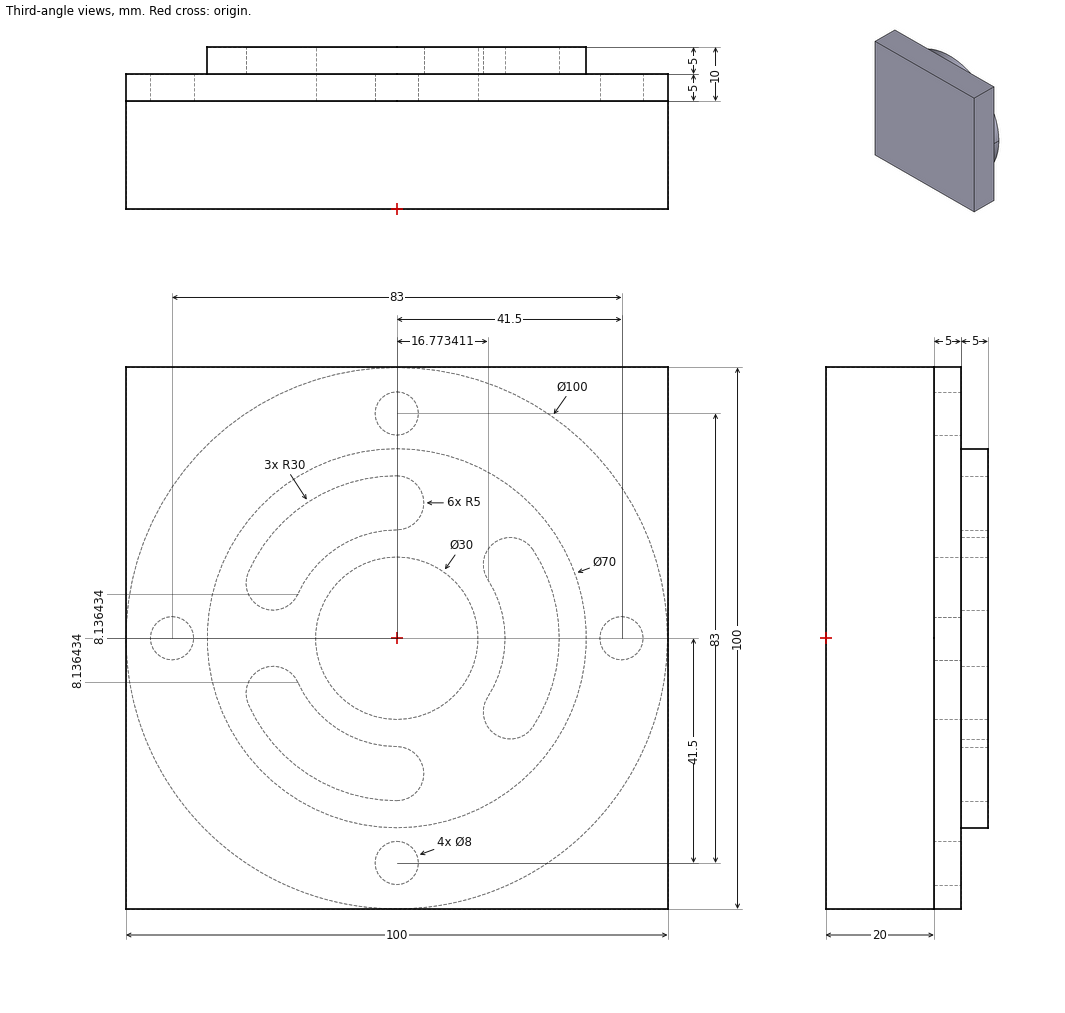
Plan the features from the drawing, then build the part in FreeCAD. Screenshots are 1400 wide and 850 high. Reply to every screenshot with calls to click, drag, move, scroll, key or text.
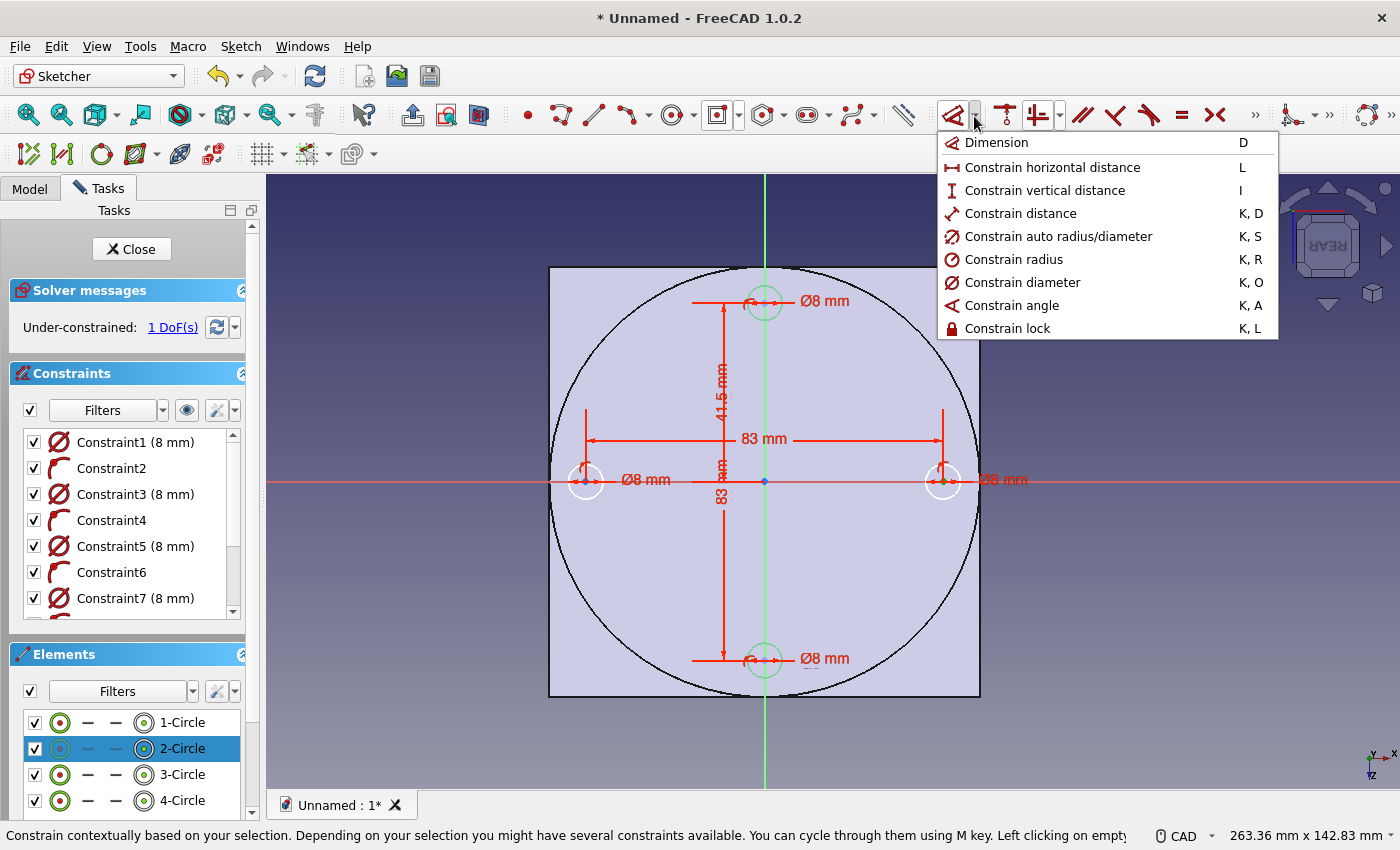
click(1108, 168)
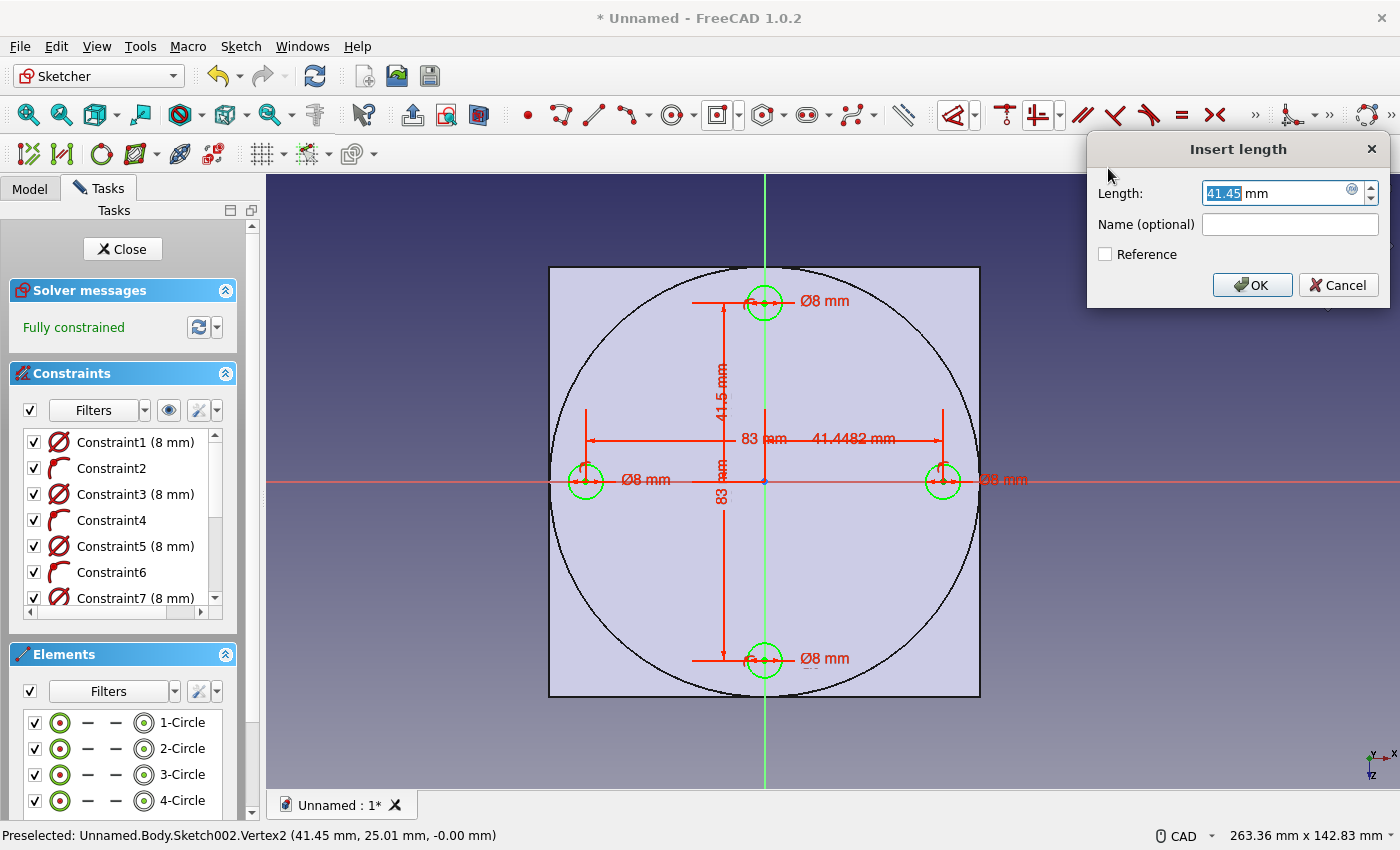
text(41.5)
key(Return)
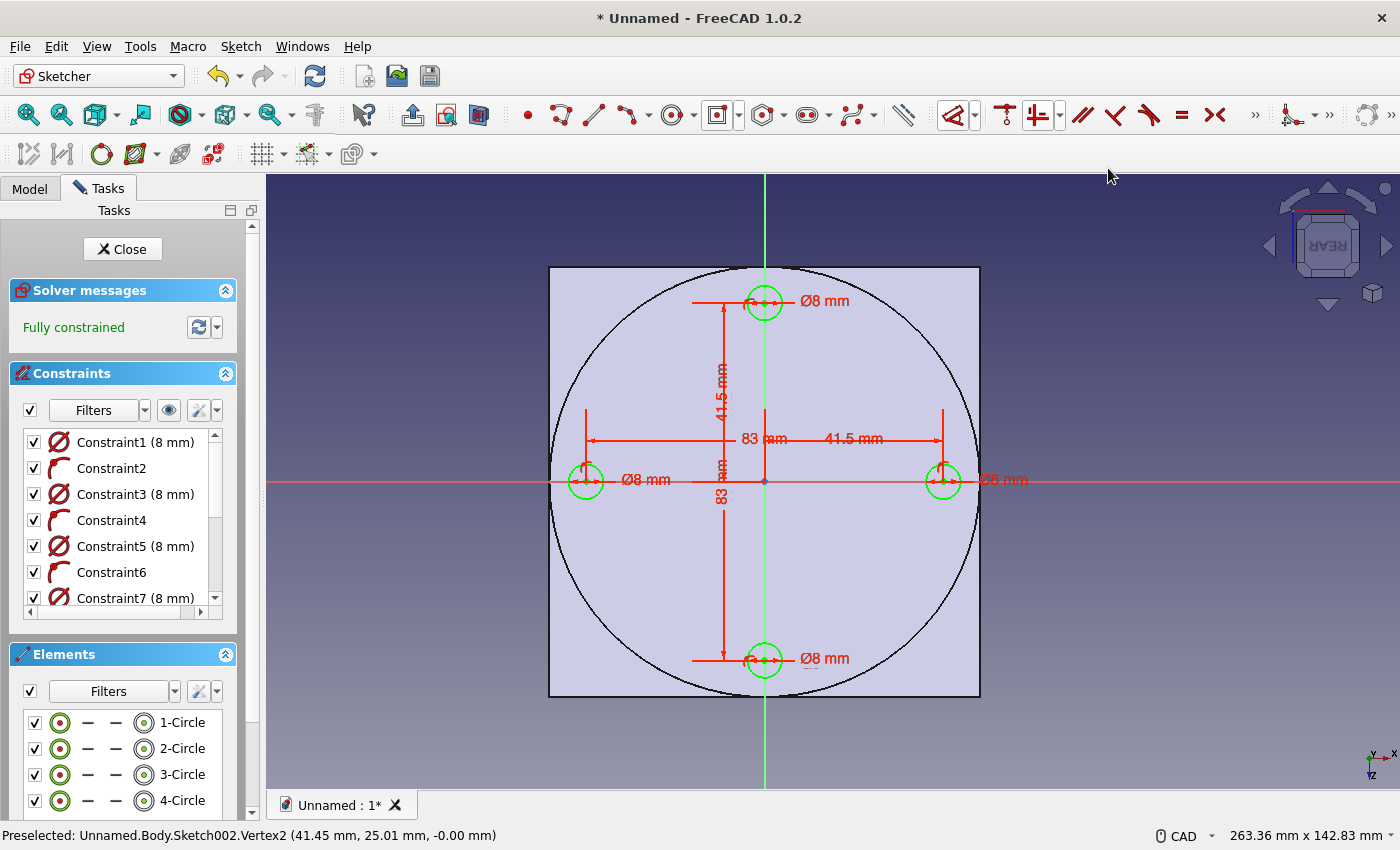
click(123, 249)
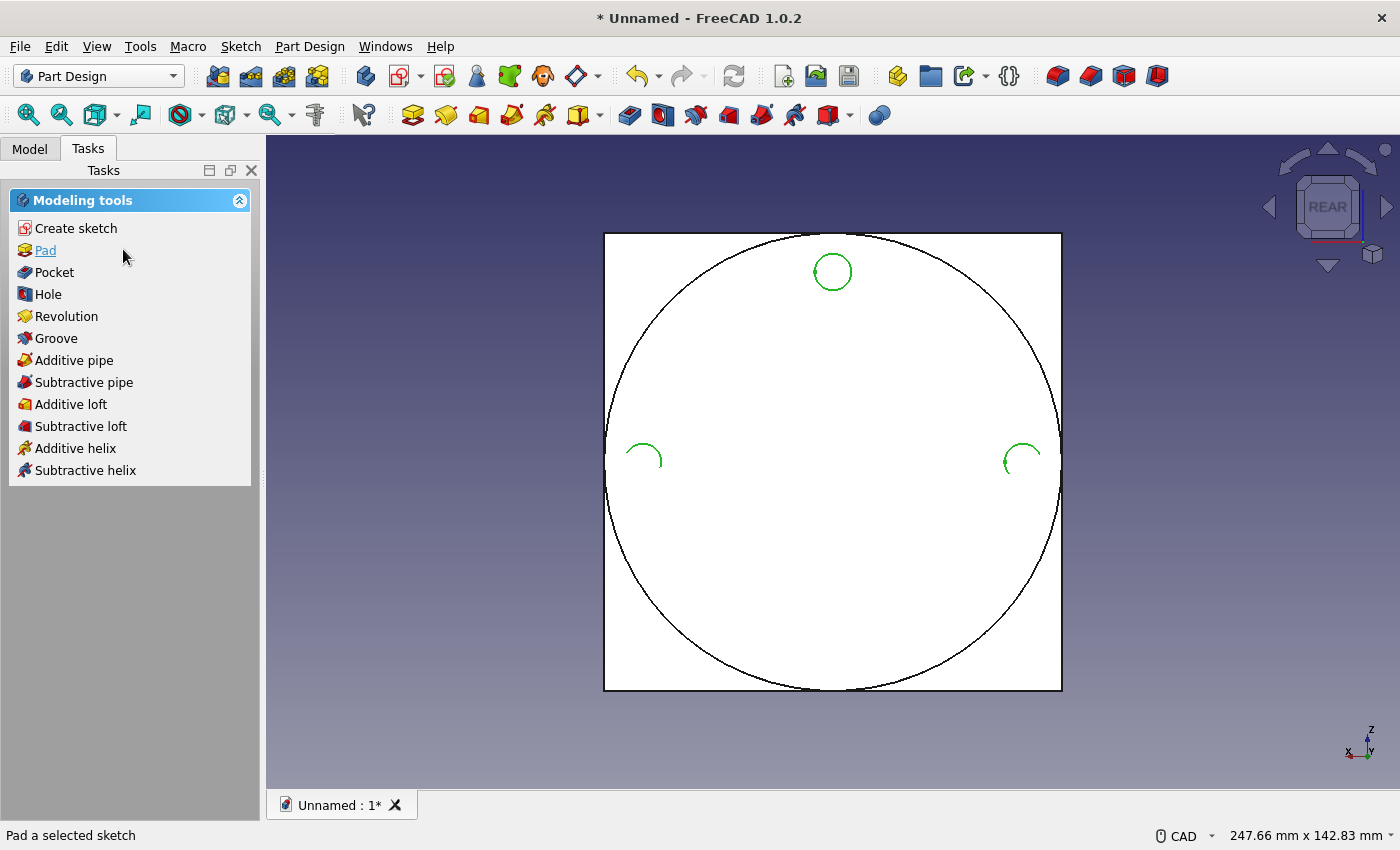
click(630, 116)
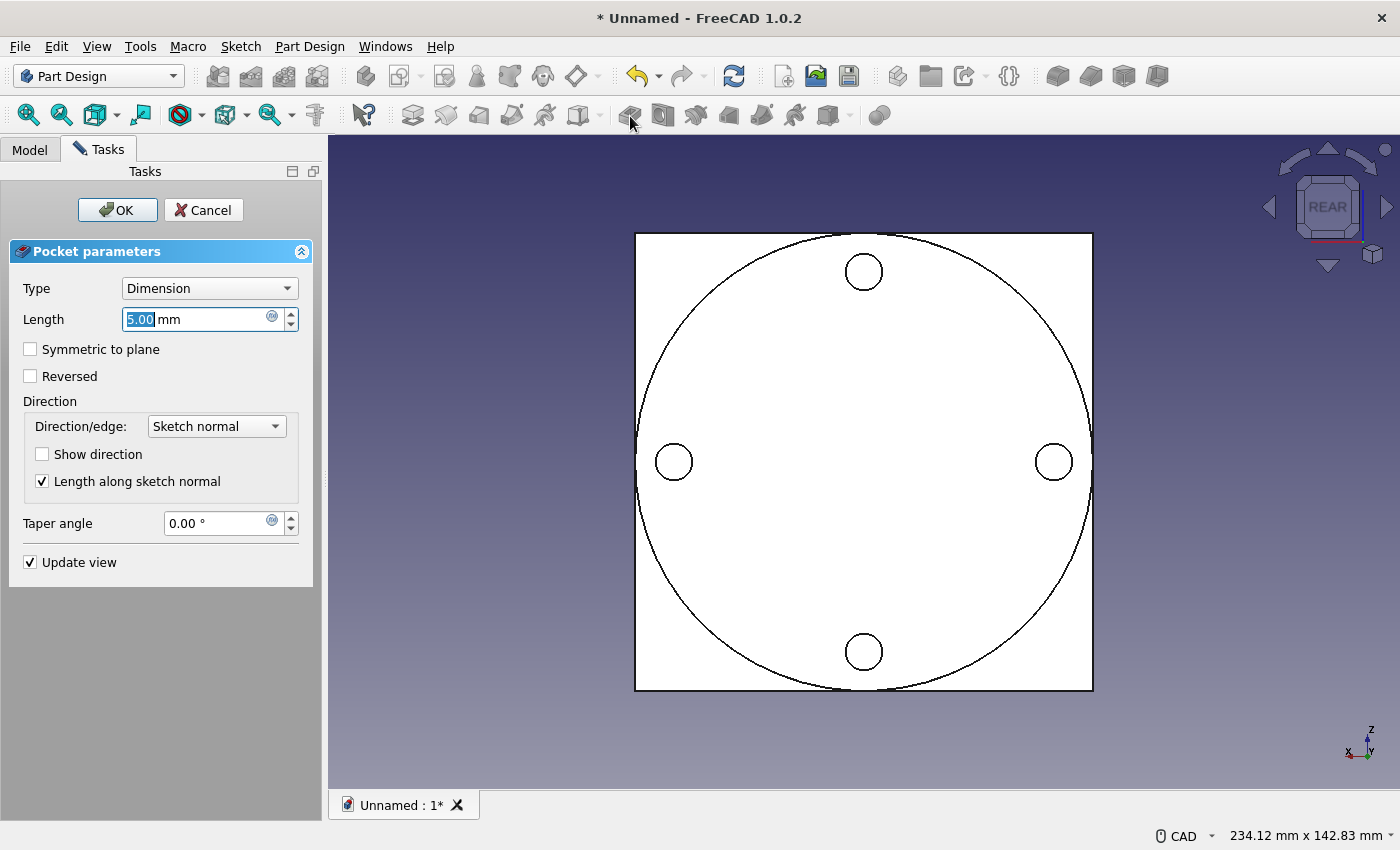
text(5)
key(Tab)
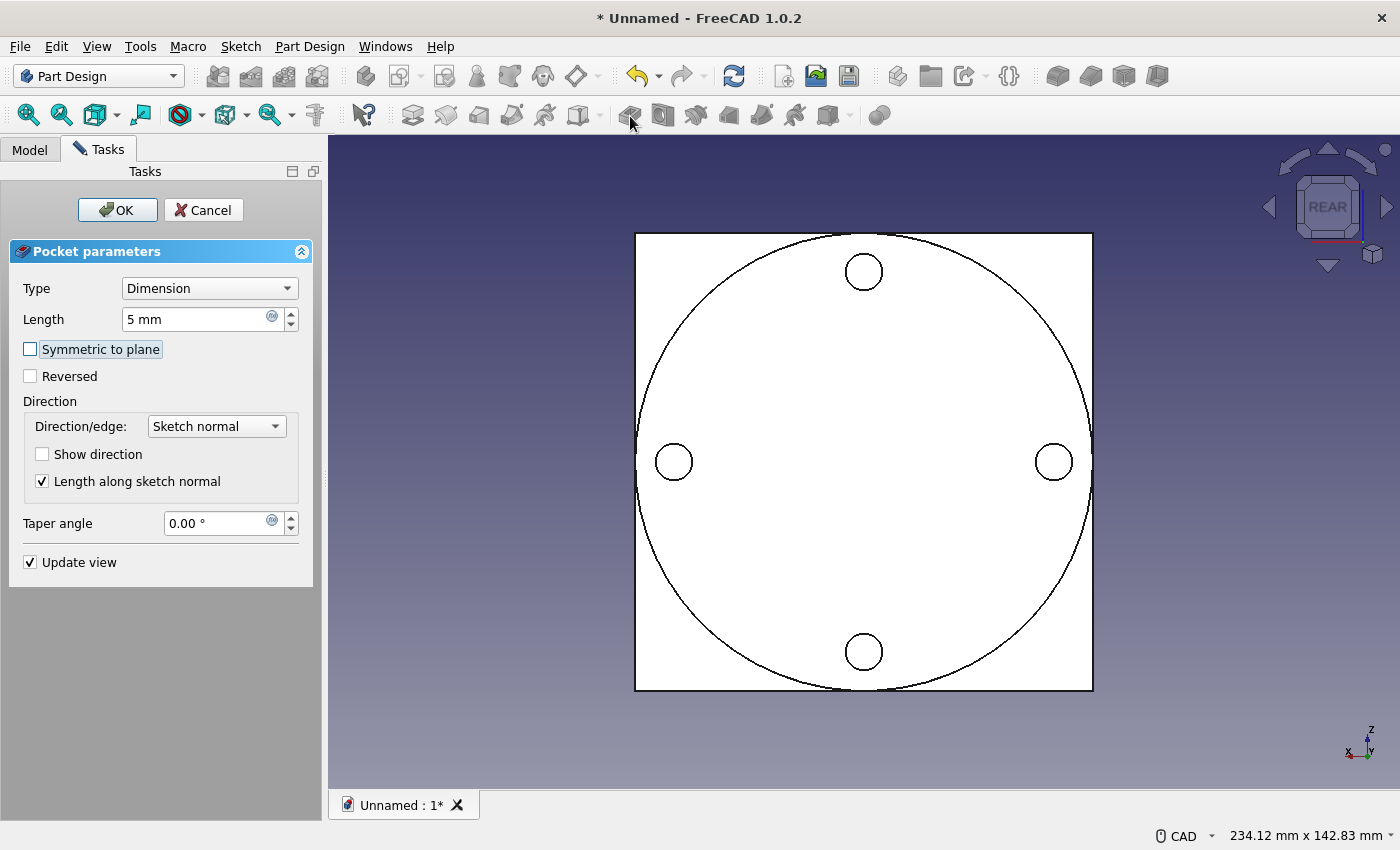
click(118, 210)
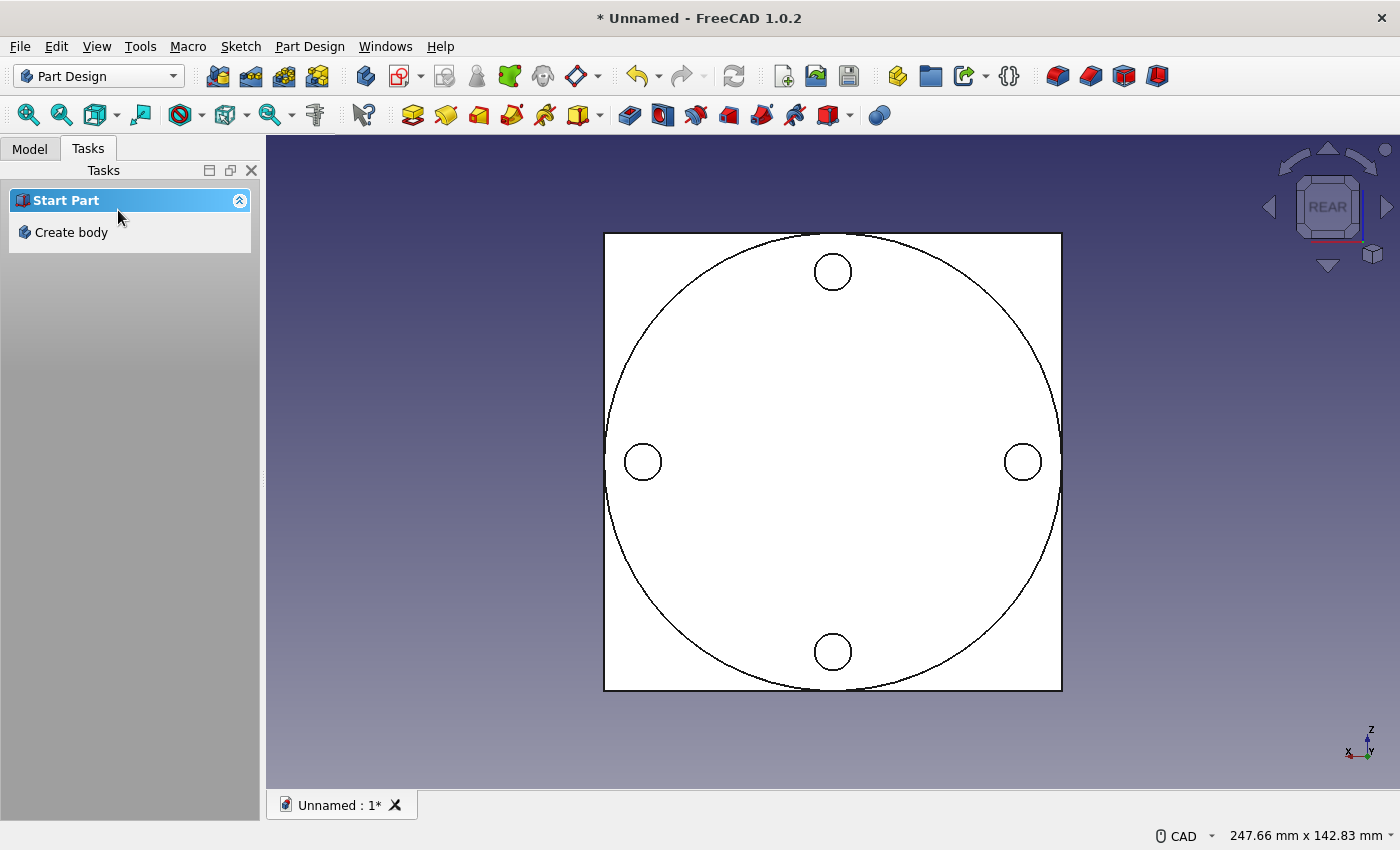
click(833, 461)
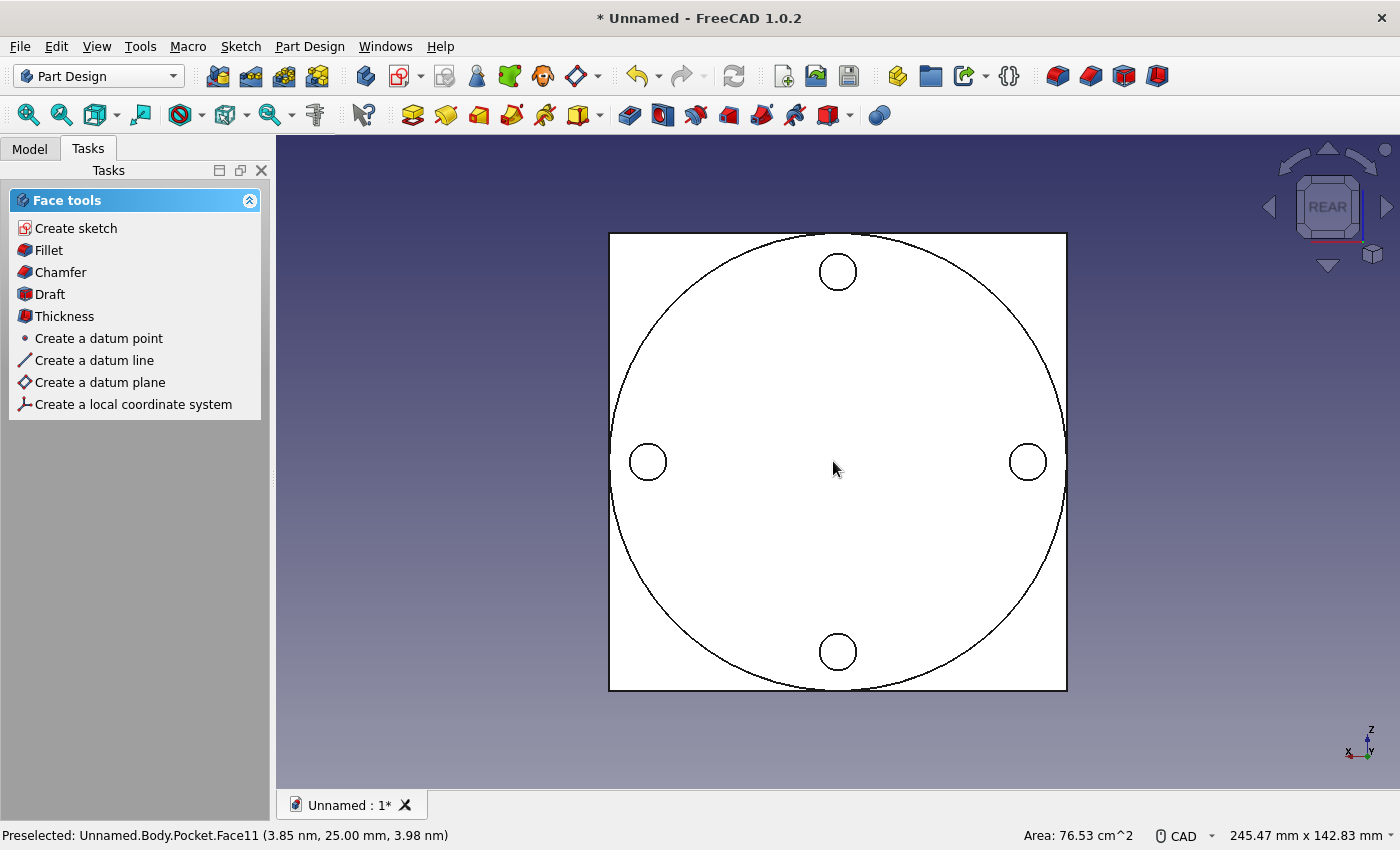
click(398, 76)